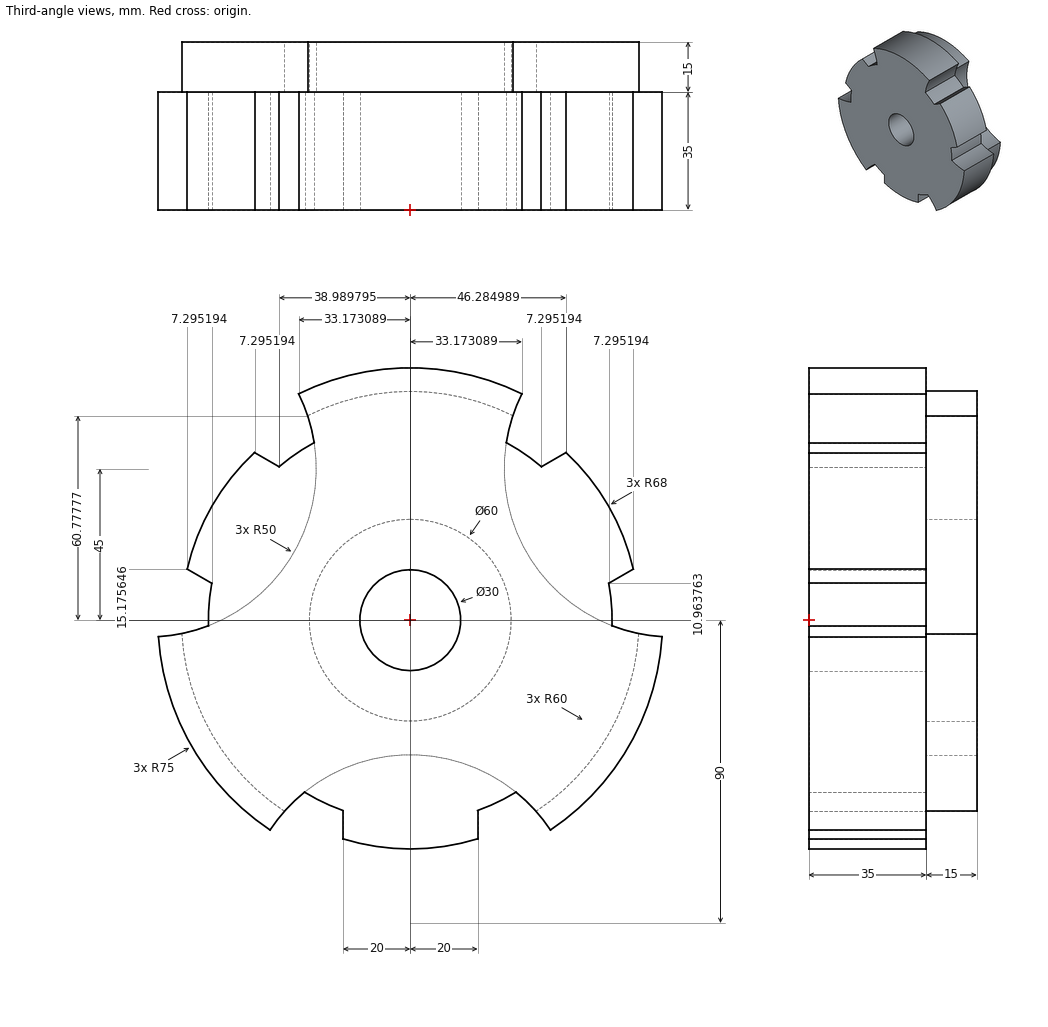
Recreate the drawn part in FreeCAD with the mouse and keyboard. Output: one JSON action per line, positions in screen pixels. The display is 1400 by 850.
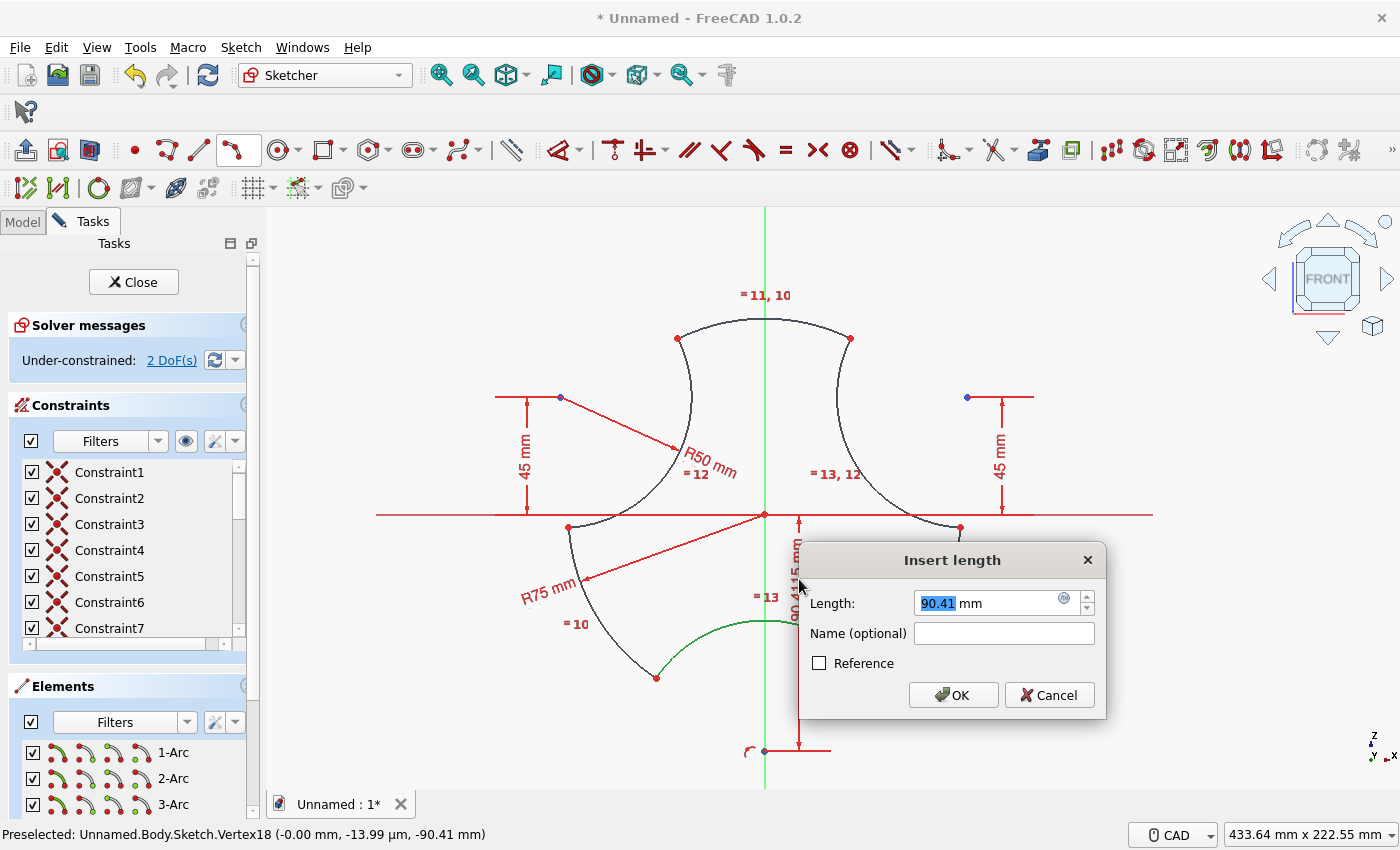
{"action": "type", "text": "90"}
{"action": "key", "text": "Return"}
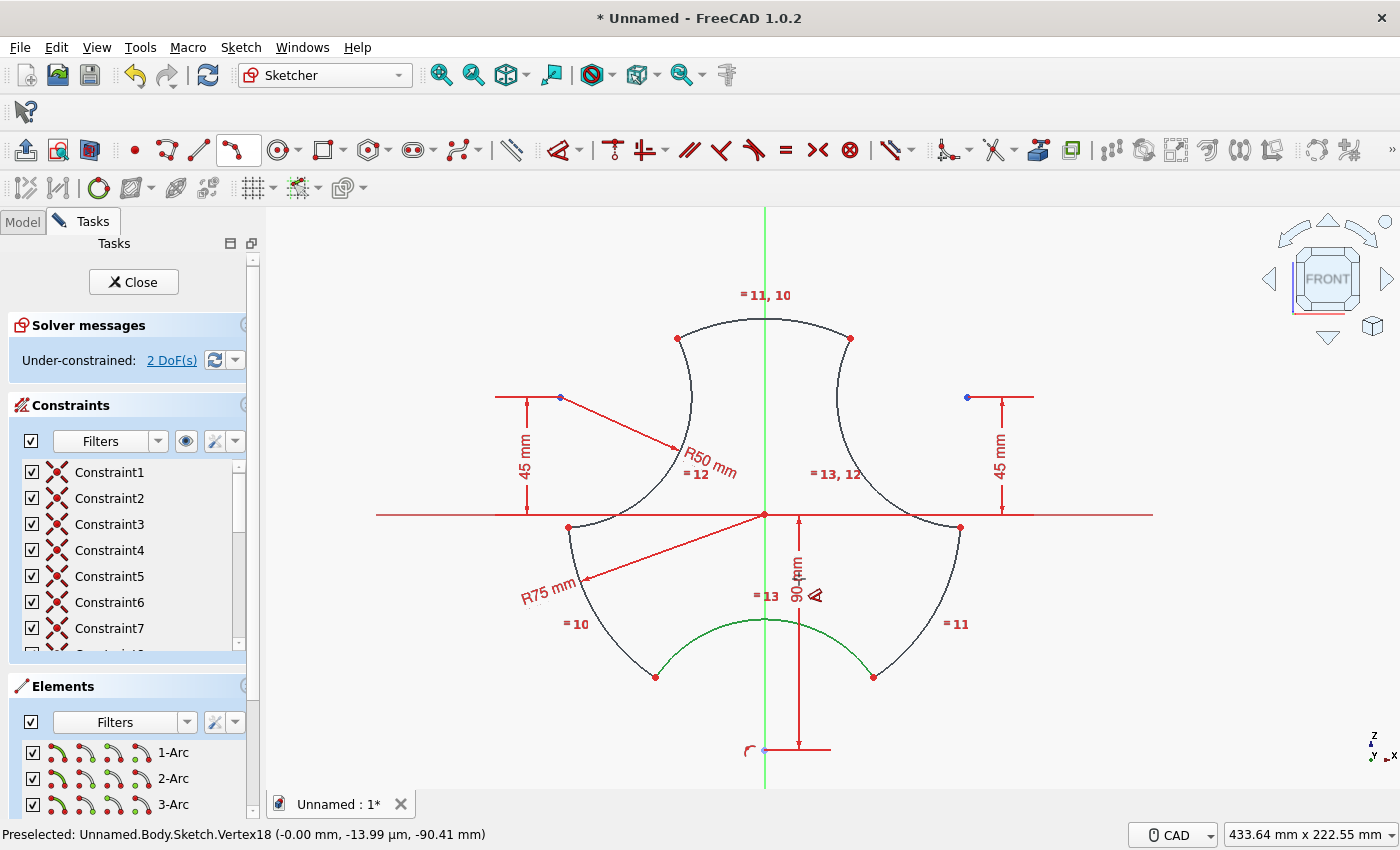
{"action": "left_click", "coordinate": [678, 339]}
{"action": "left_click", "coordinate": [721, 305]}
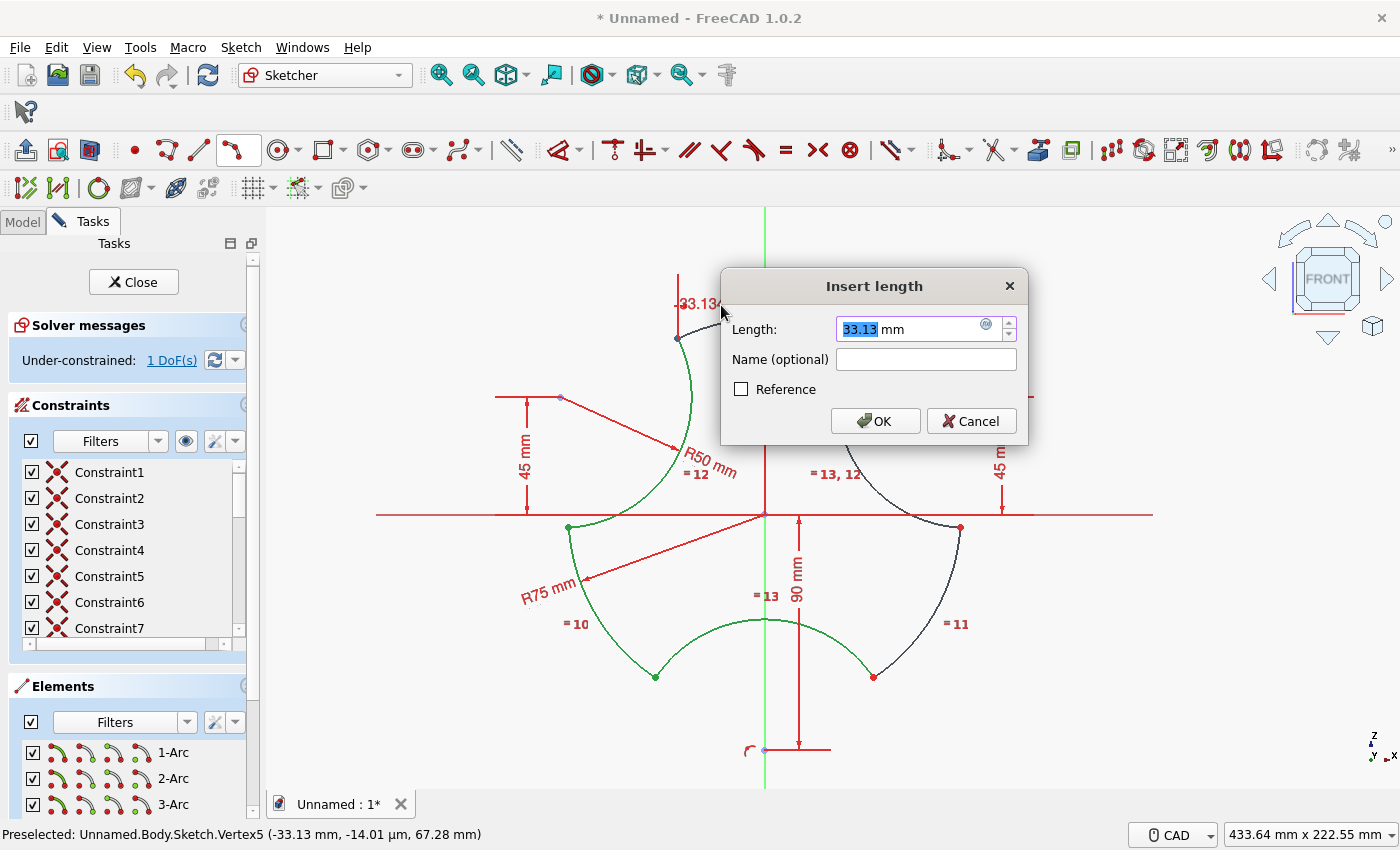
{"action": "type", "text": "33.173089"}
{"action": "key", "text": "Return"}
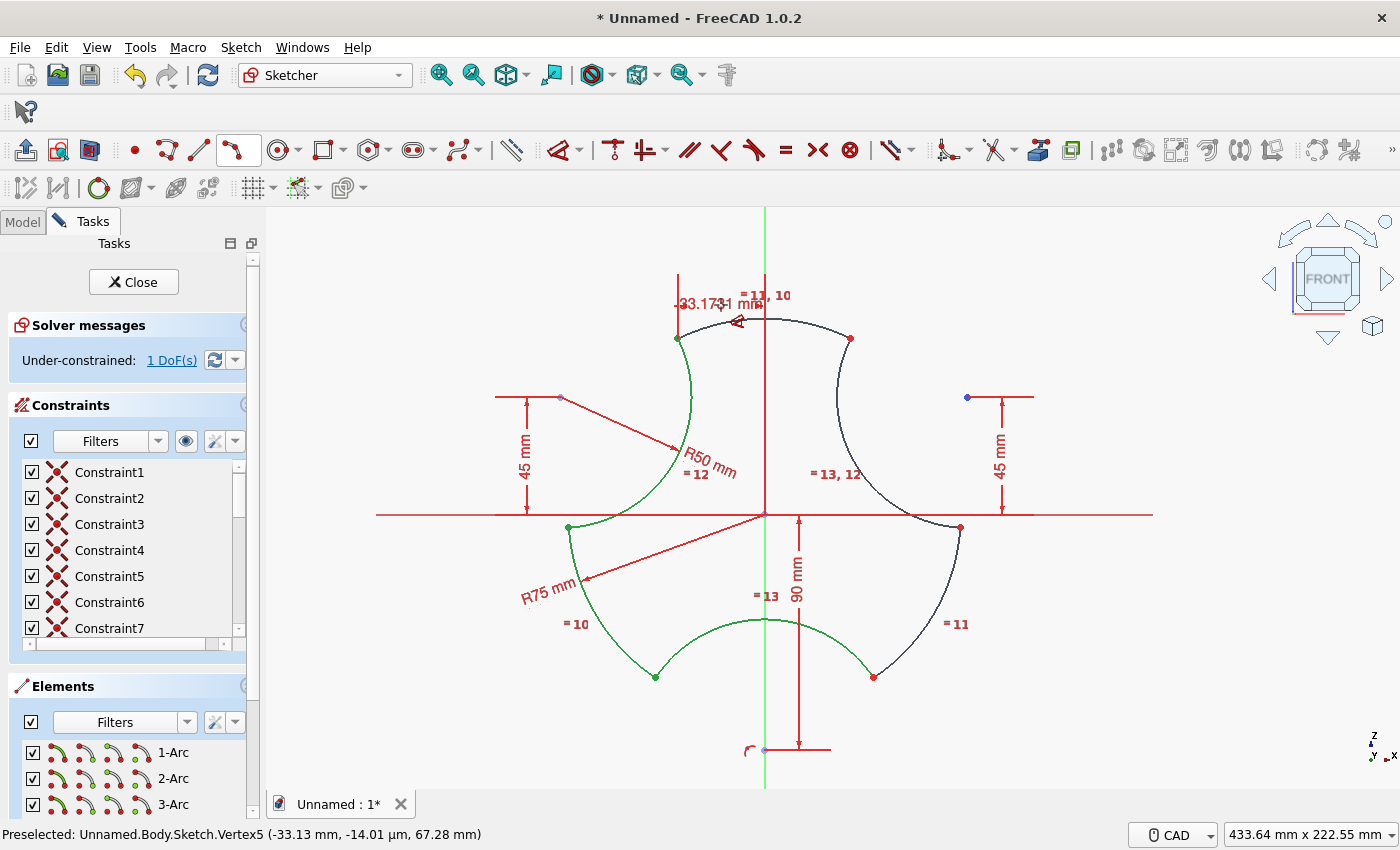
{"action": "left_click", "coordinate": [851, 339]}
{"action": "left_click", "coordinate": [808, 305]}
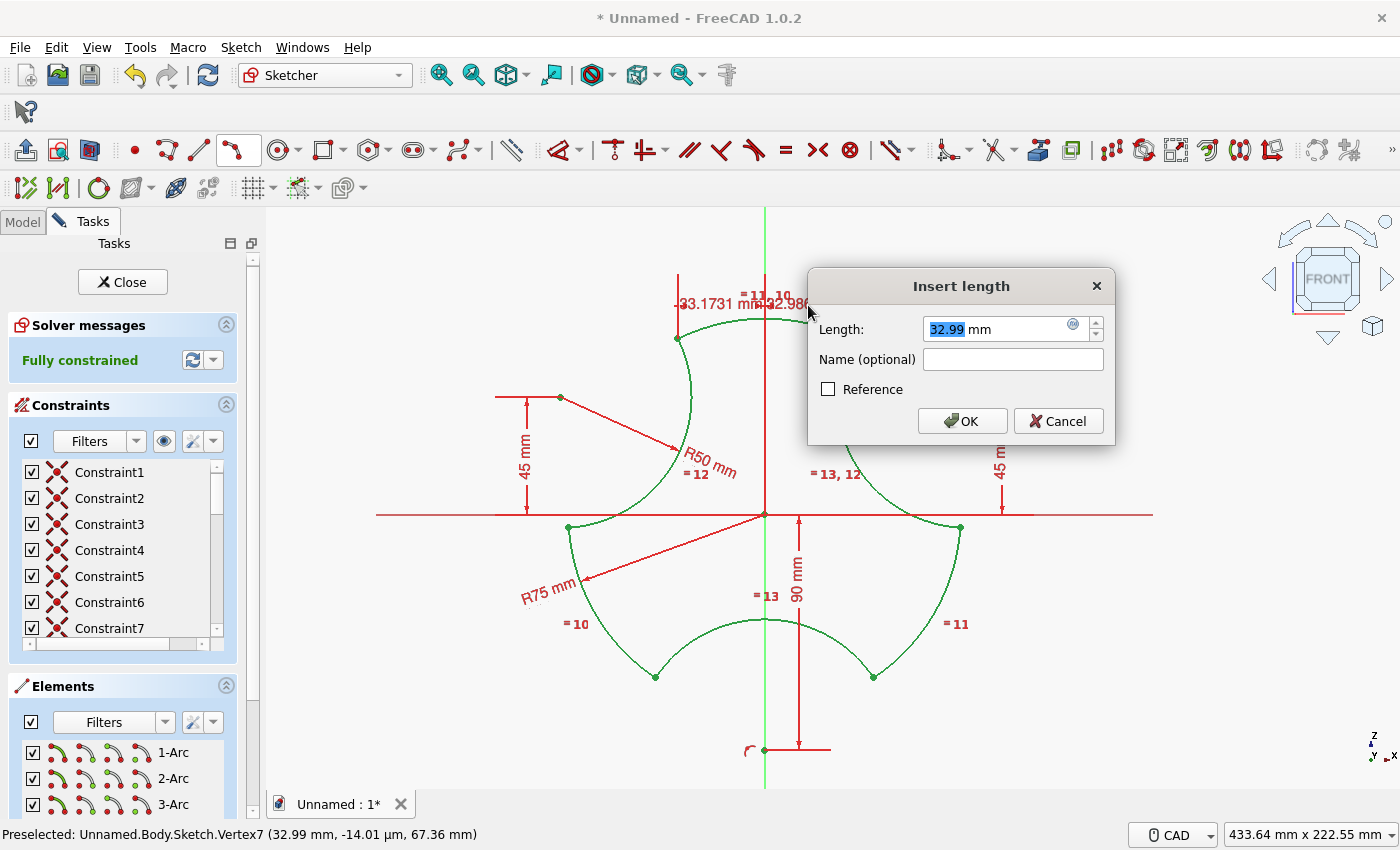
{"action": "type", "text": "33.173089"}
{"action": "key", "text": "Return"}
{"action": "key", "text": "Escape"}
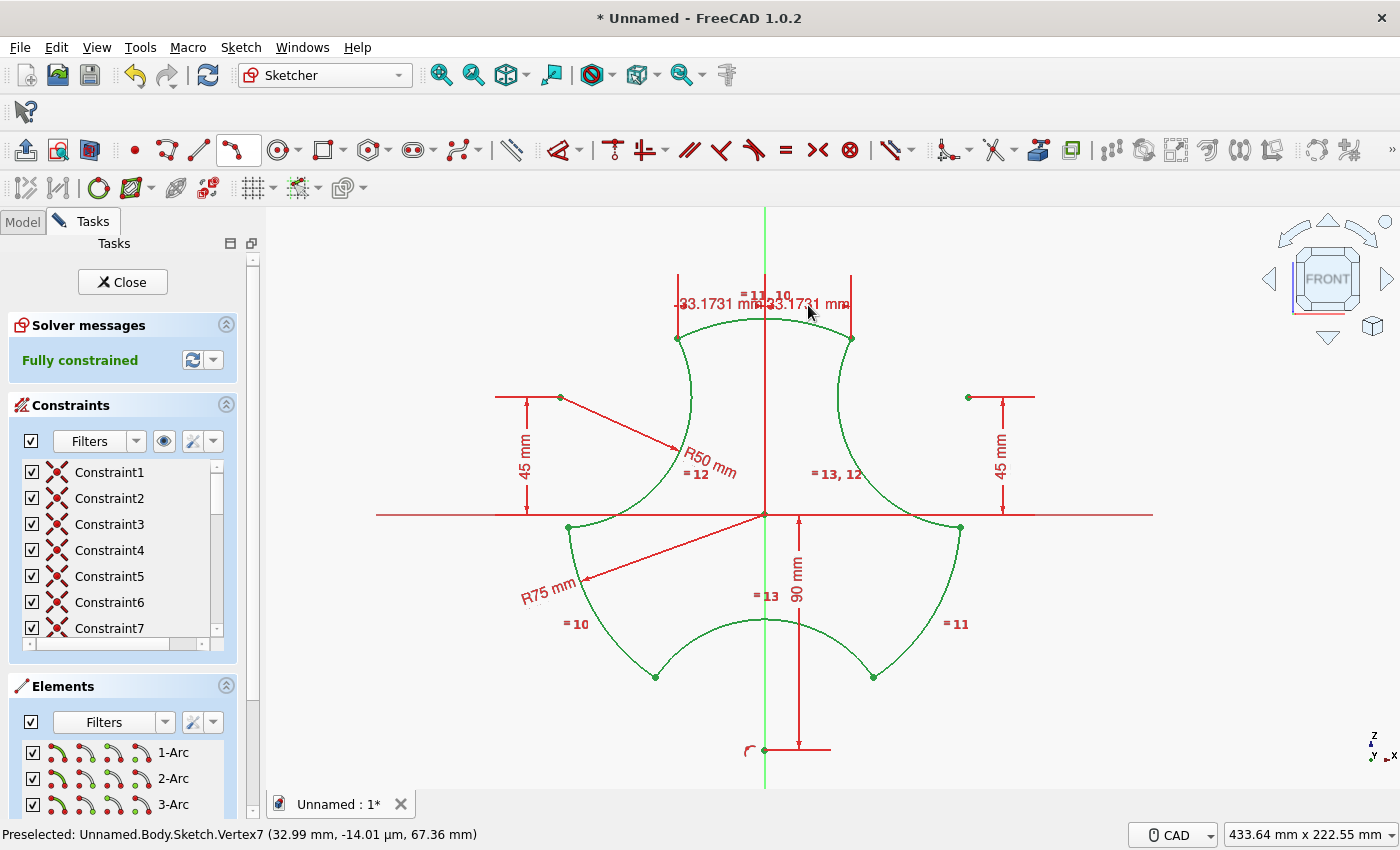
{"action": "left_click", "coordinate": [123, 282]}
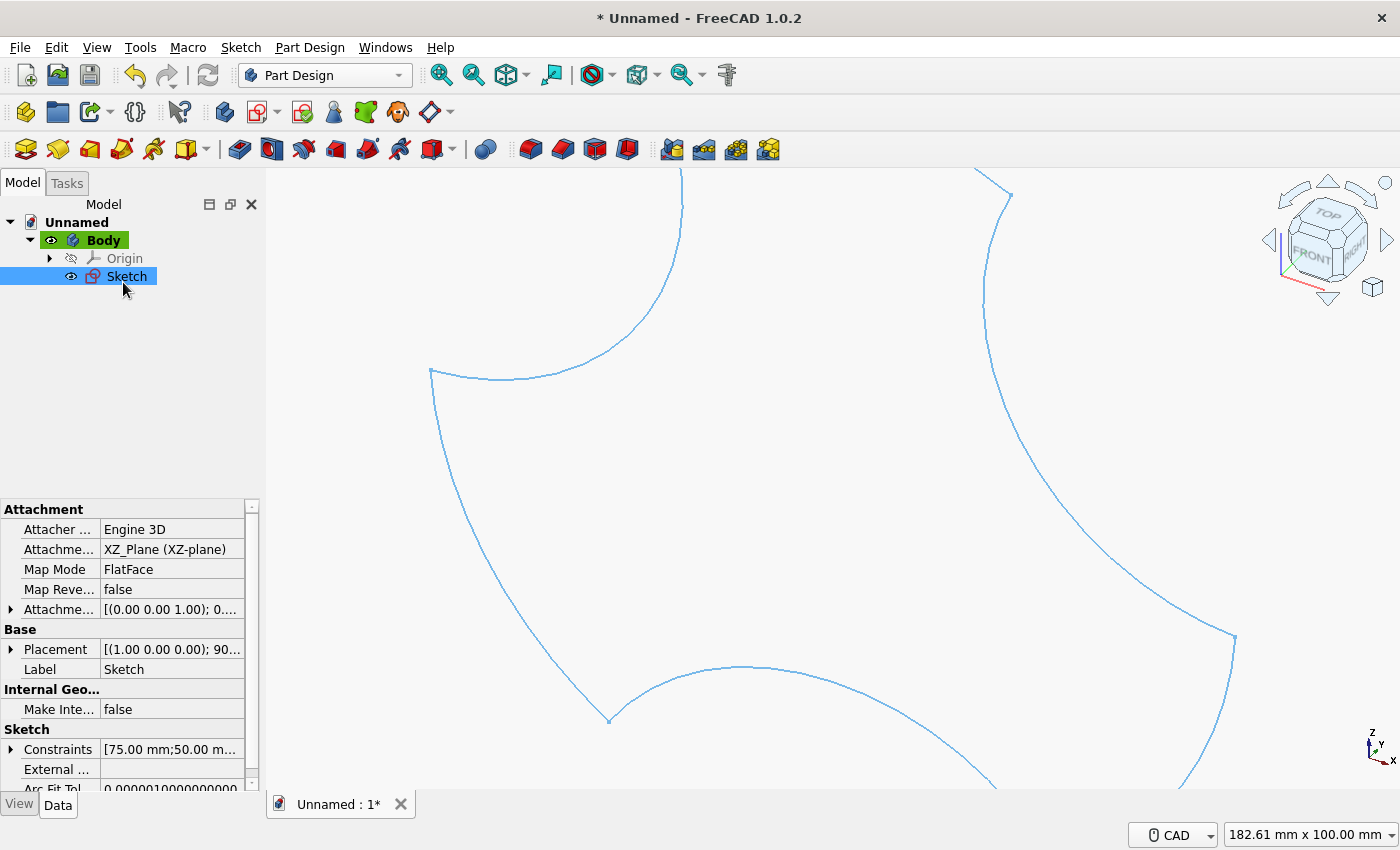
{"action": "left_click", "coordinate": [26, 150]}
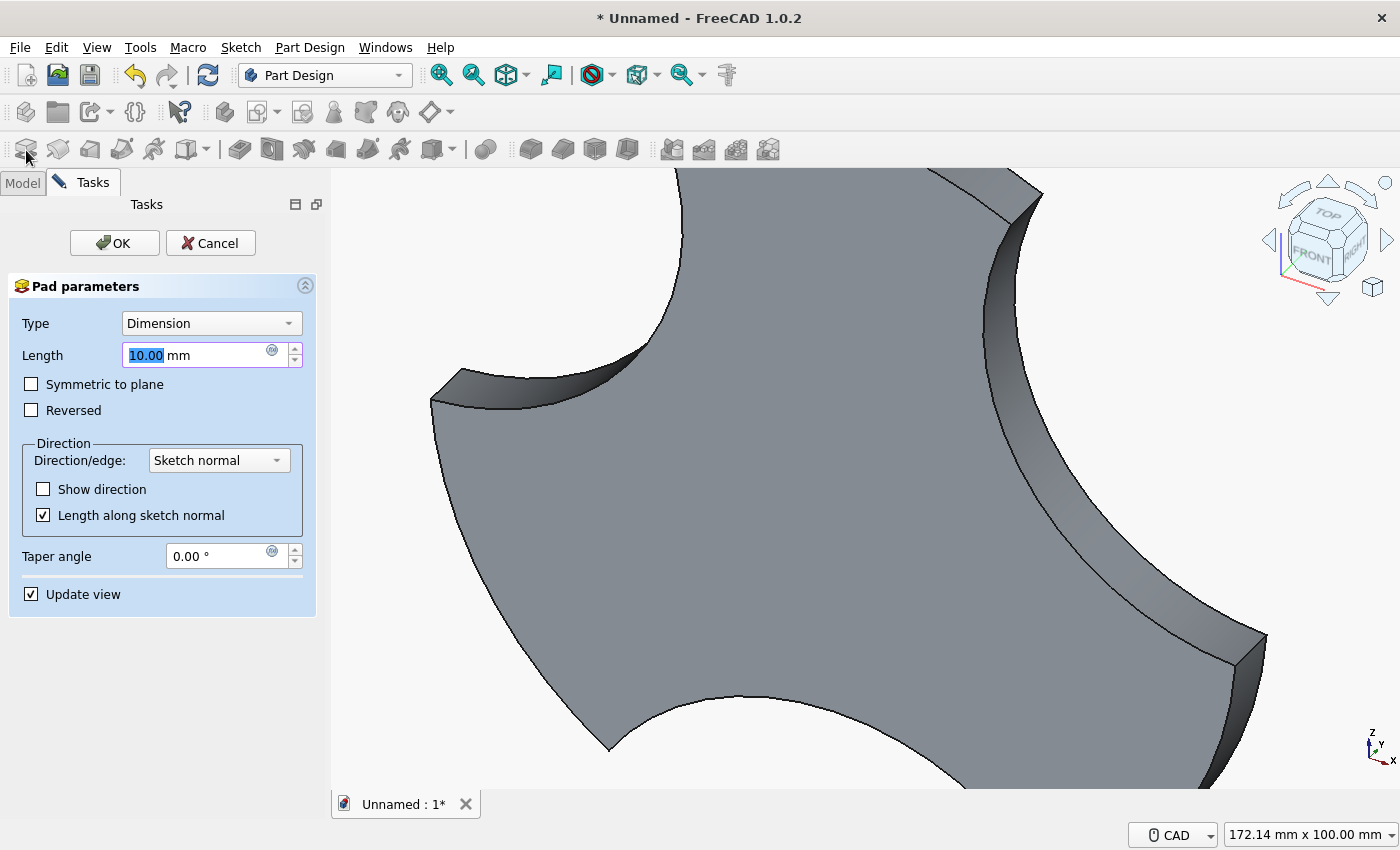
{"action": "type", "text": "35"}
{"action": "key", "text": "Tab"}